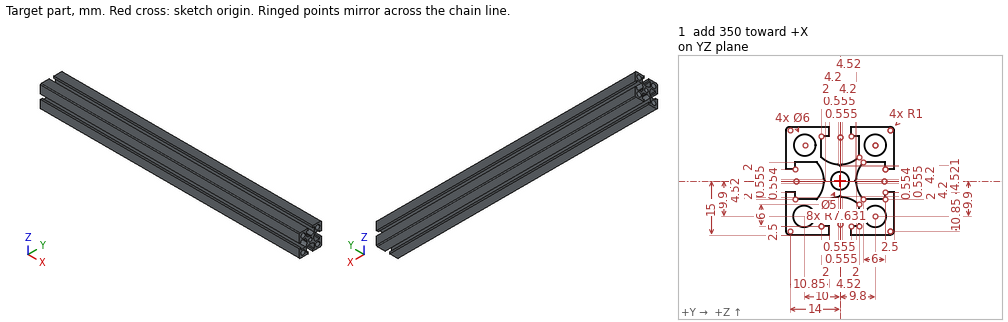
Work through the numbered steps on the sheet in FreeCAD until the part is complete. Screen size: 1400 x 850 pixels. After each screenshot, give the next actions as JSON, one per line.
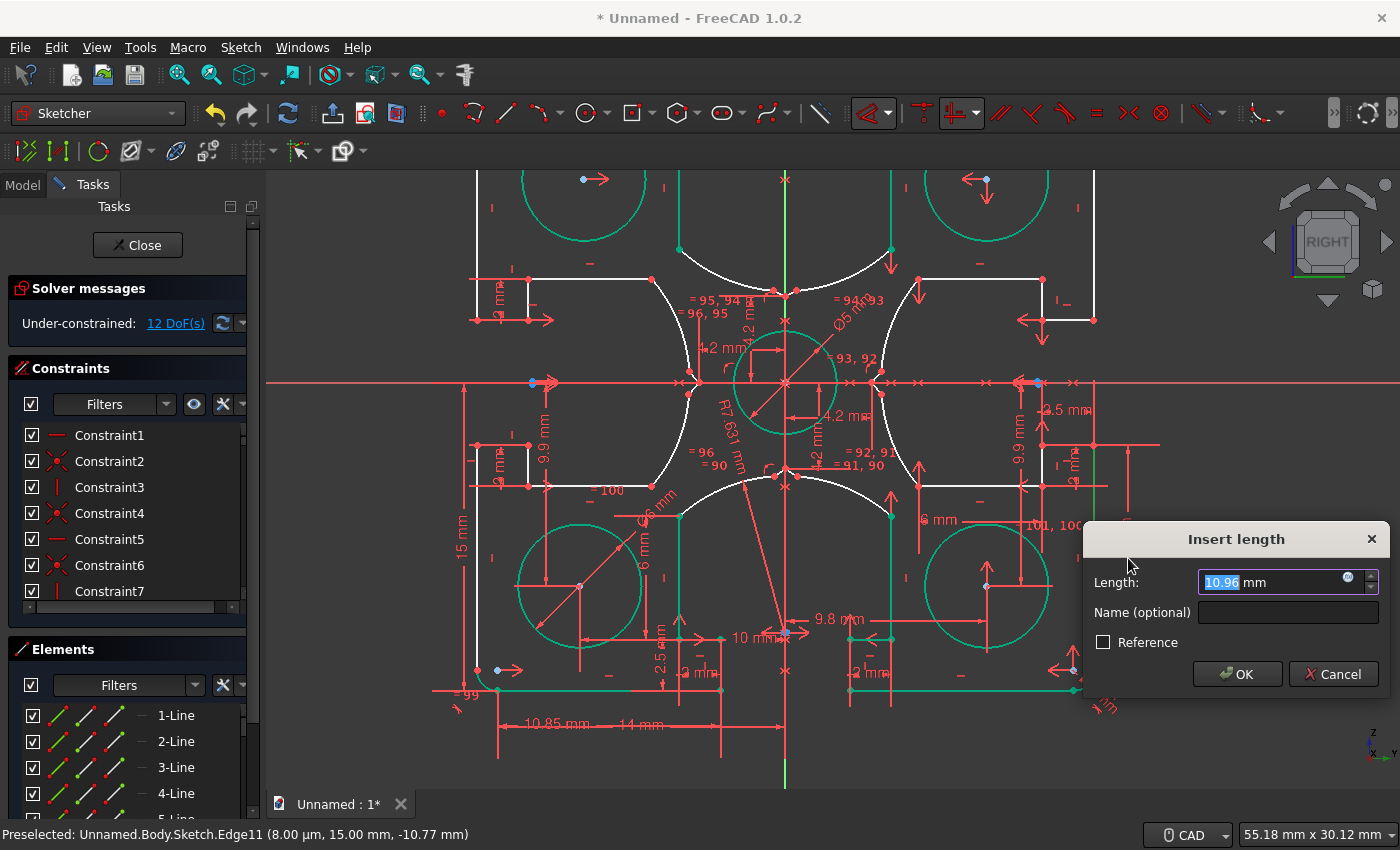
{"action": "type", "text": "10.85"}
{"action": "key", "text": "Return"}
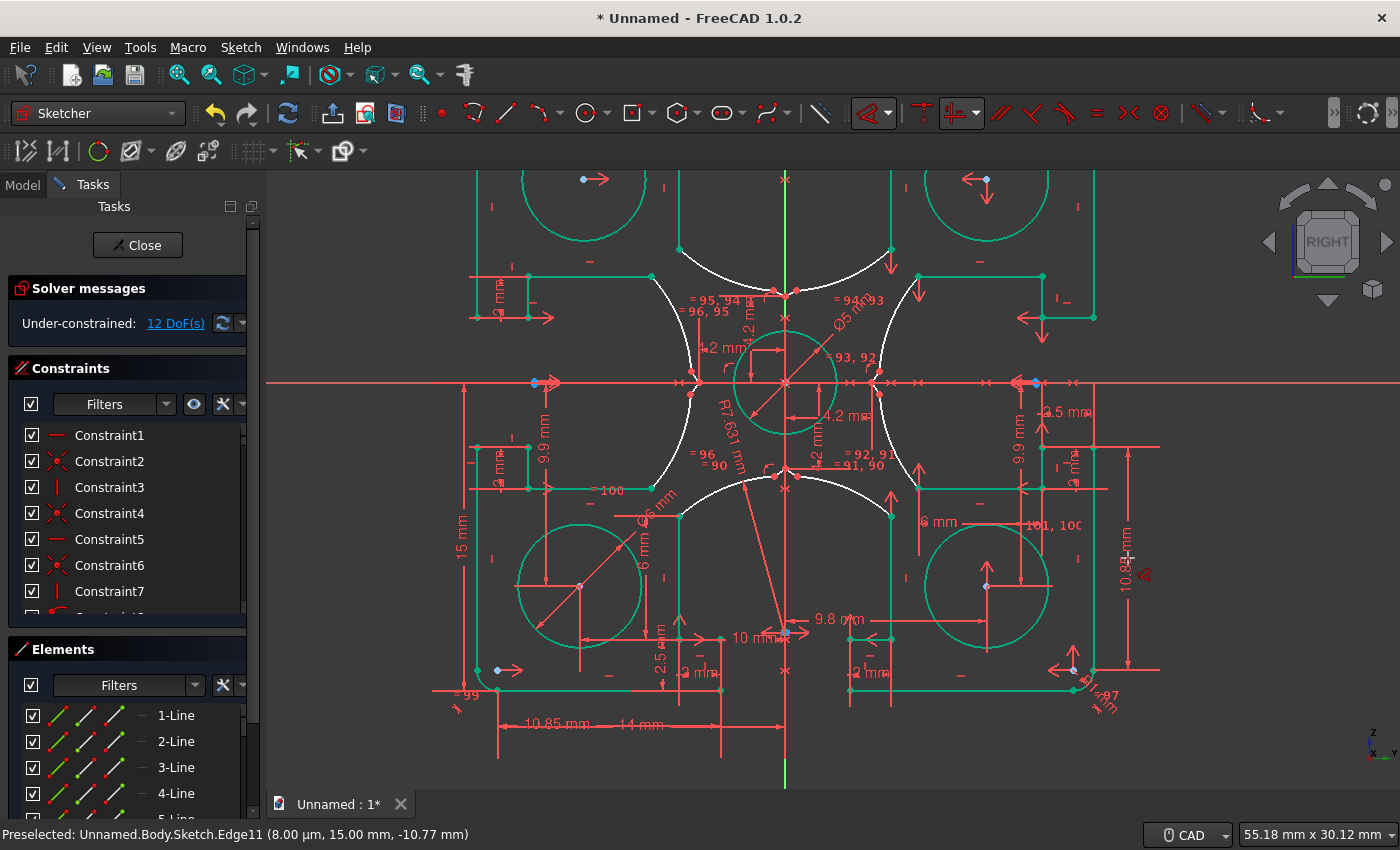
{"action": "left_click", "coordinate": [774, 476]}
{"action": "left_click", "coordinate": [740, 462]}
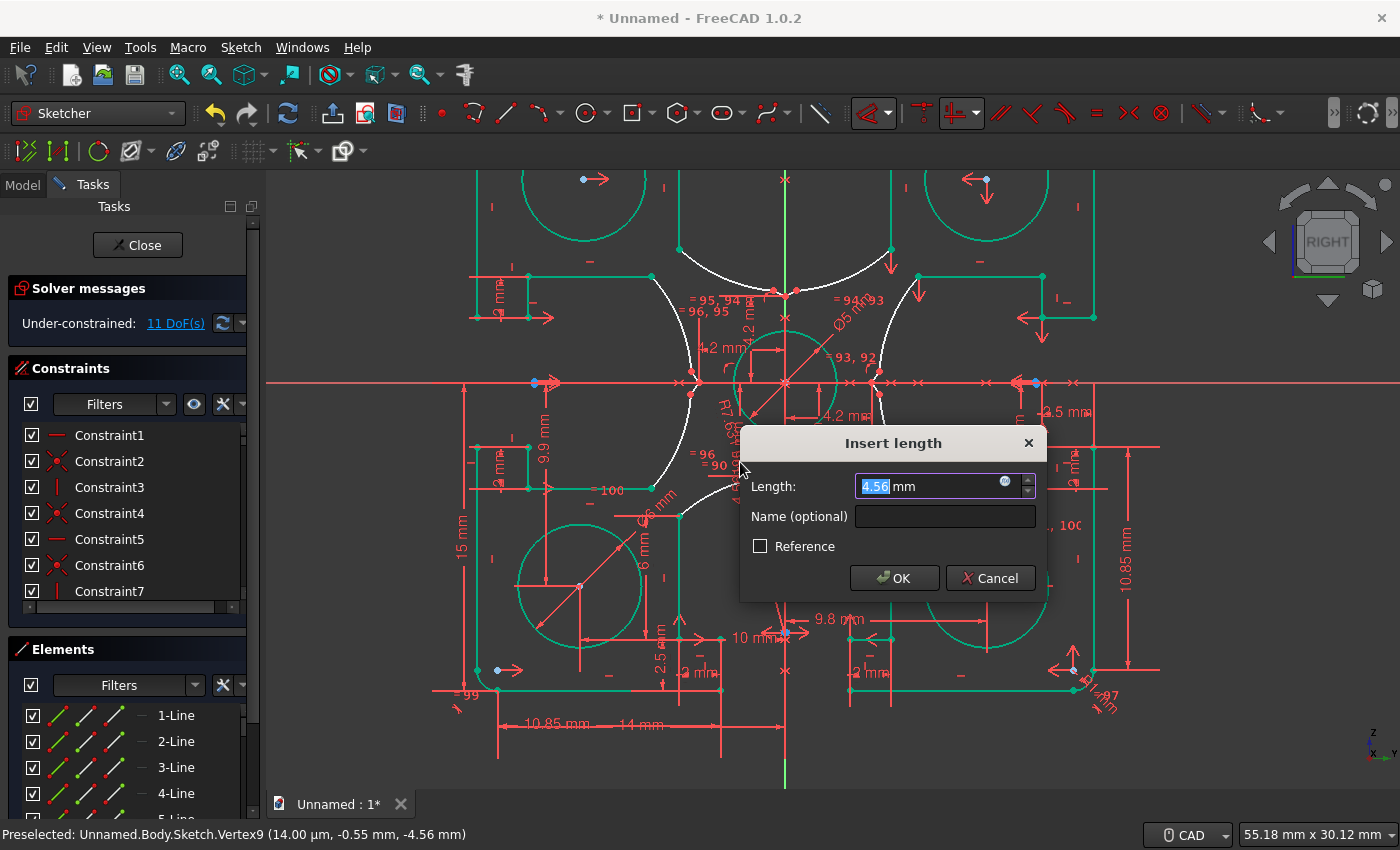
{"action": "type", "text": "4.52"}
{"action": "key", "text": "Return"}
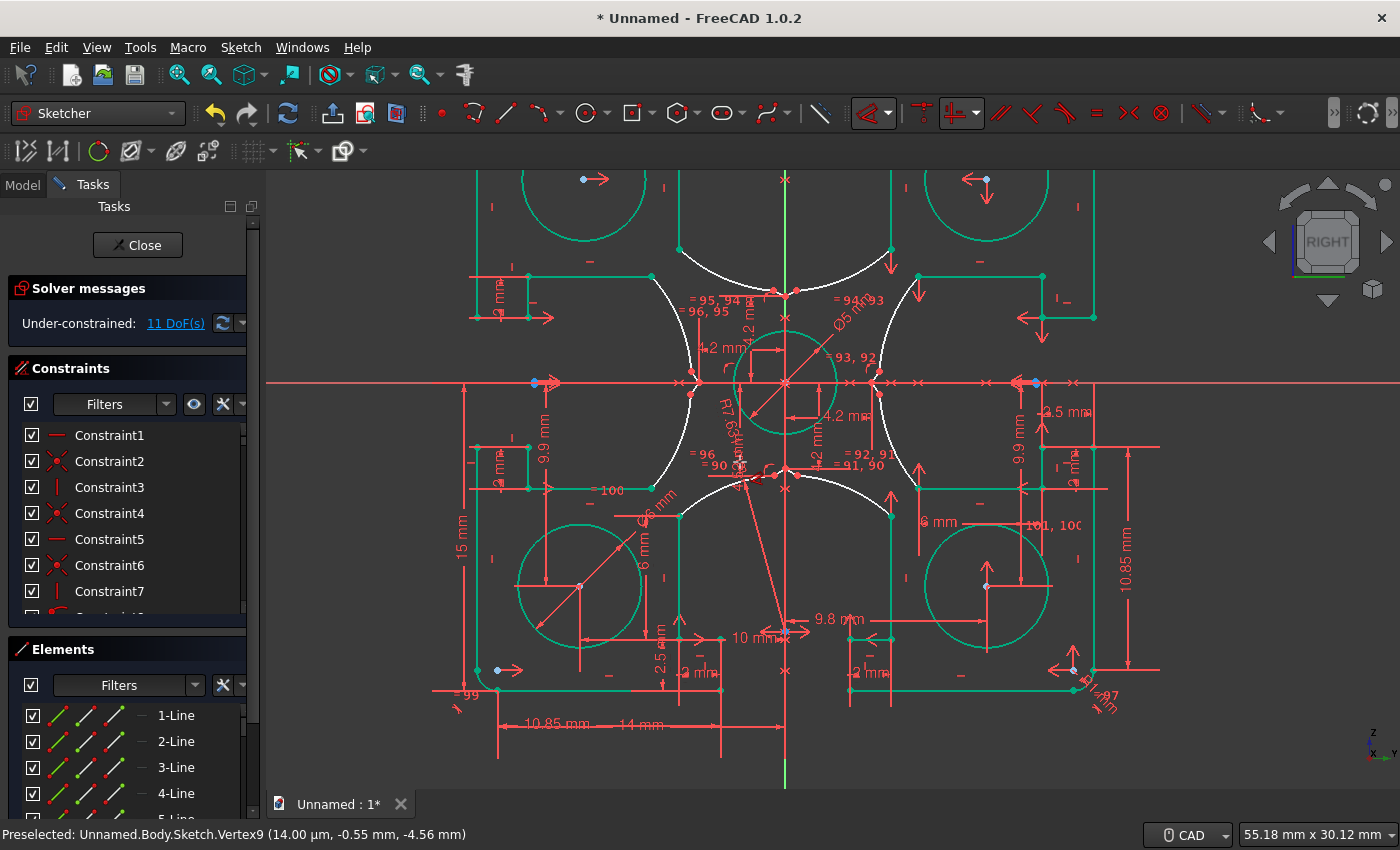
{"action": "left_click", "coordinate": [880, 394]}
{"action": "left_click", "coordinate": [854, 349]}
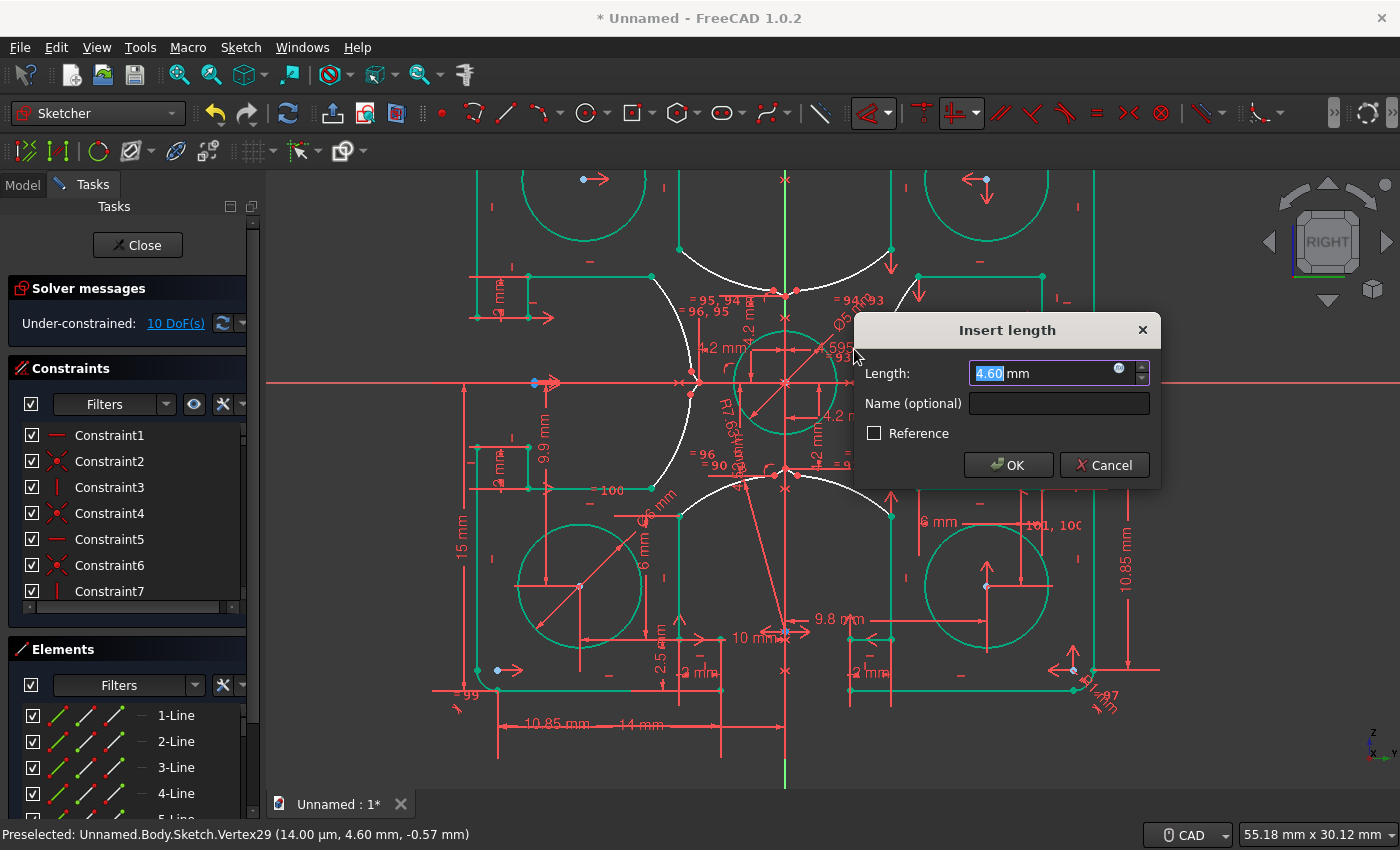
{"action": "type", "text": "4.52"}
{"action": "key", "text": "Return"}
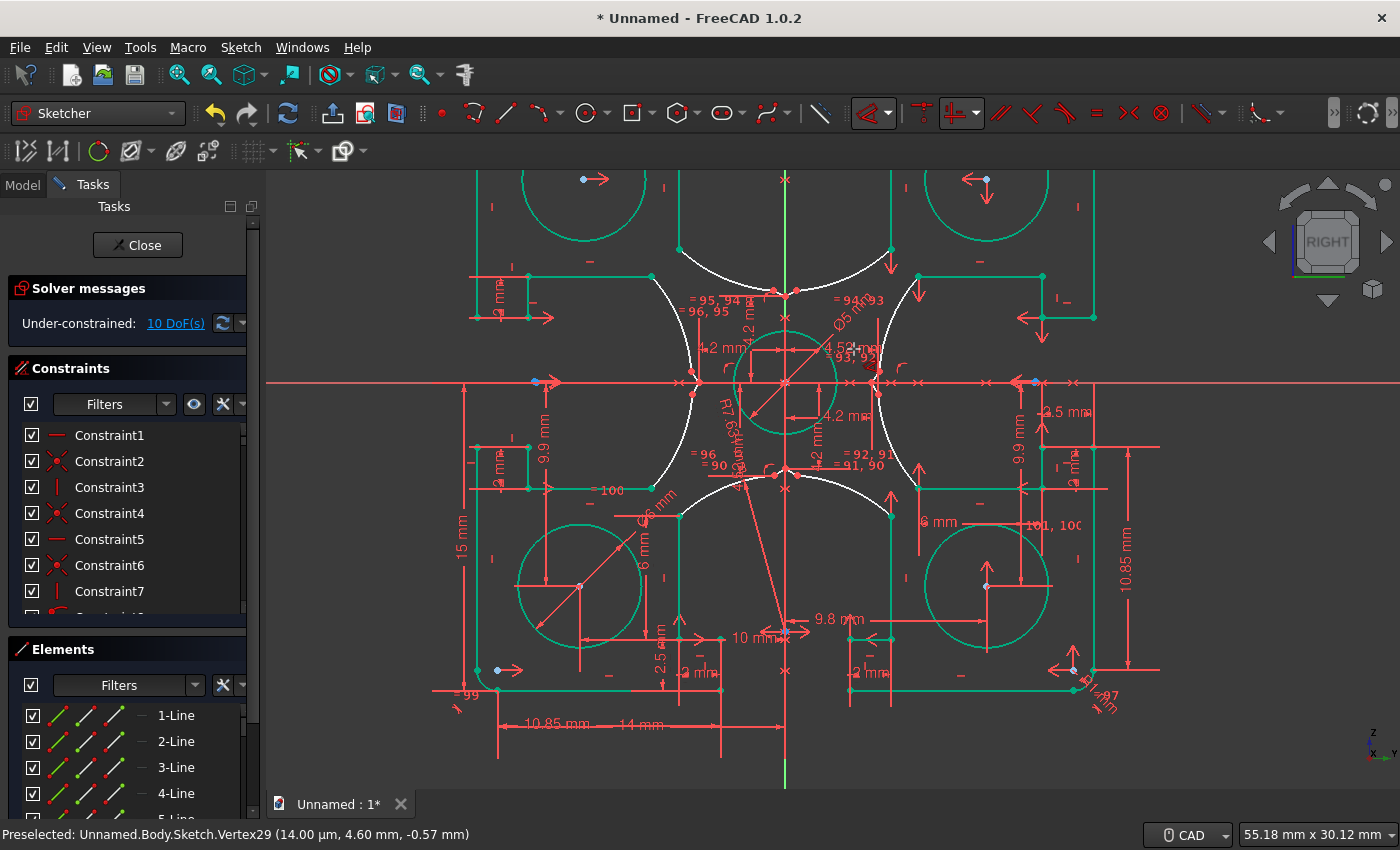
{"action": "left_click", "coordinate": [879, 372]}
{"action": "left_click", "coordinate": [854, 290]}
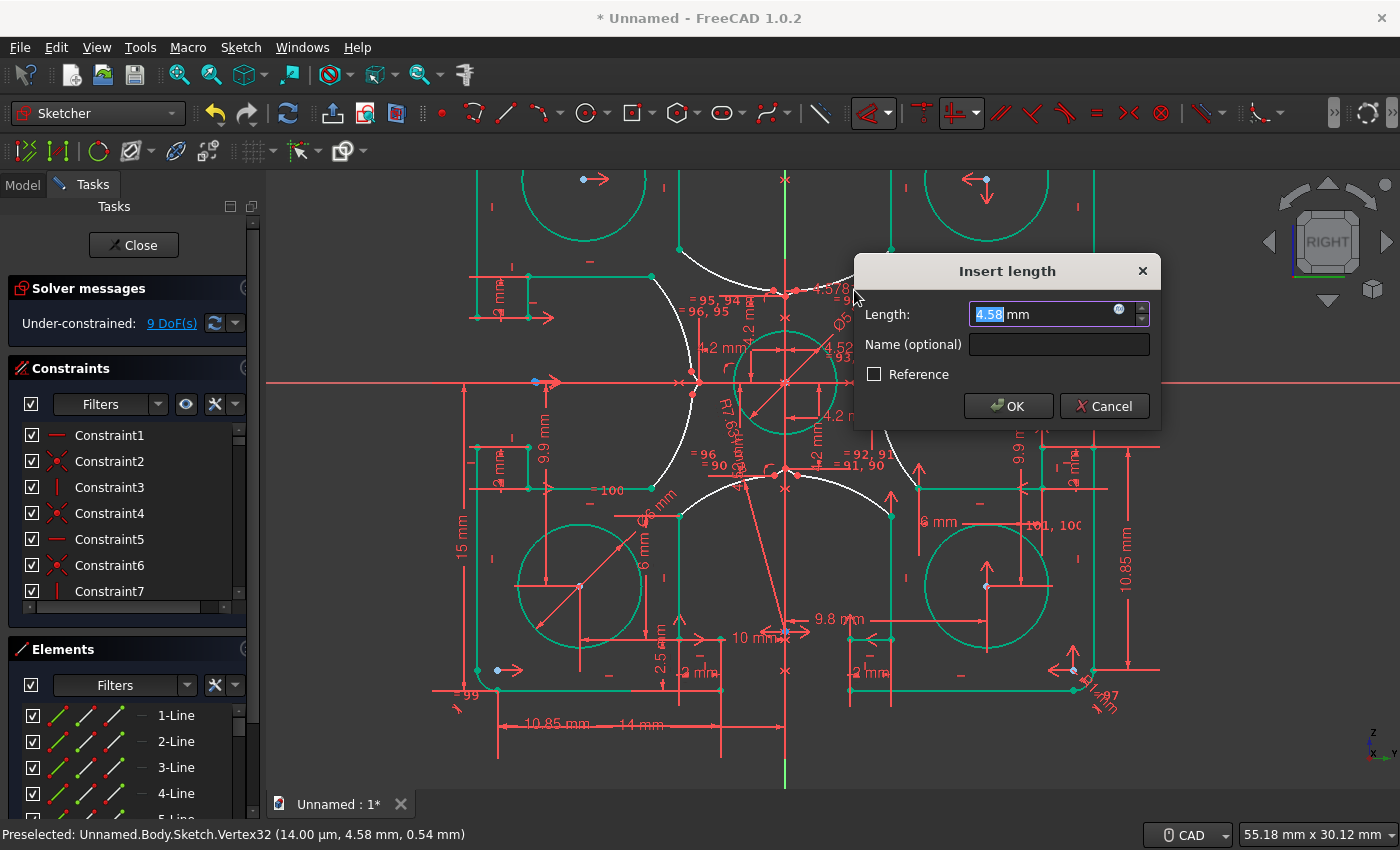
{"action": "type", "text": "4.52"}
{"action": "key", "text": "Return"}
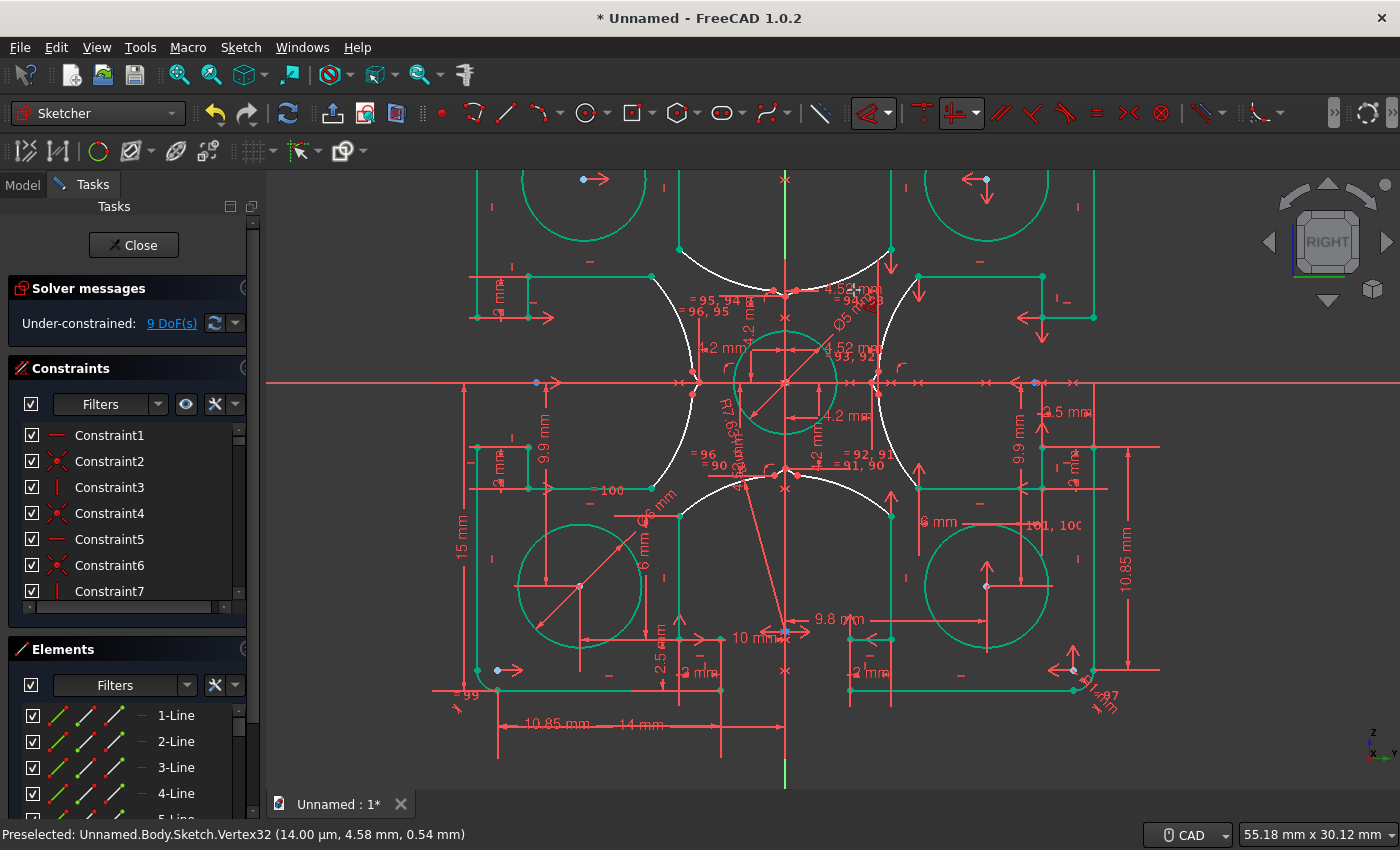
{"action": "scroll", "coordinate": [774, 476], "scroll_direction": "up", "scroll_amount": 7}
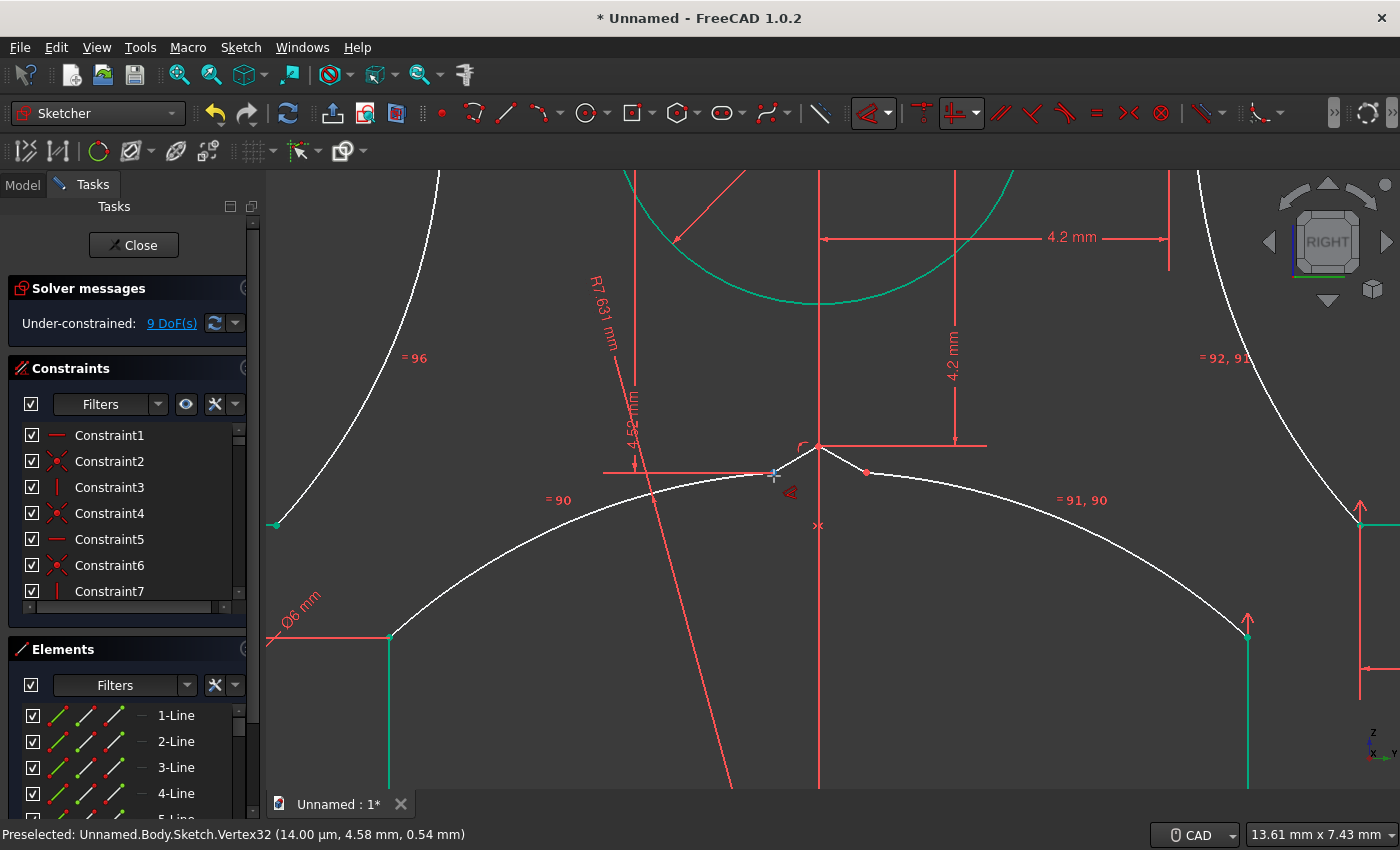
{"action": "left_click", "coordinate": [773, 473]}
{"action": "left_click", "coordinate": [796, 507]}